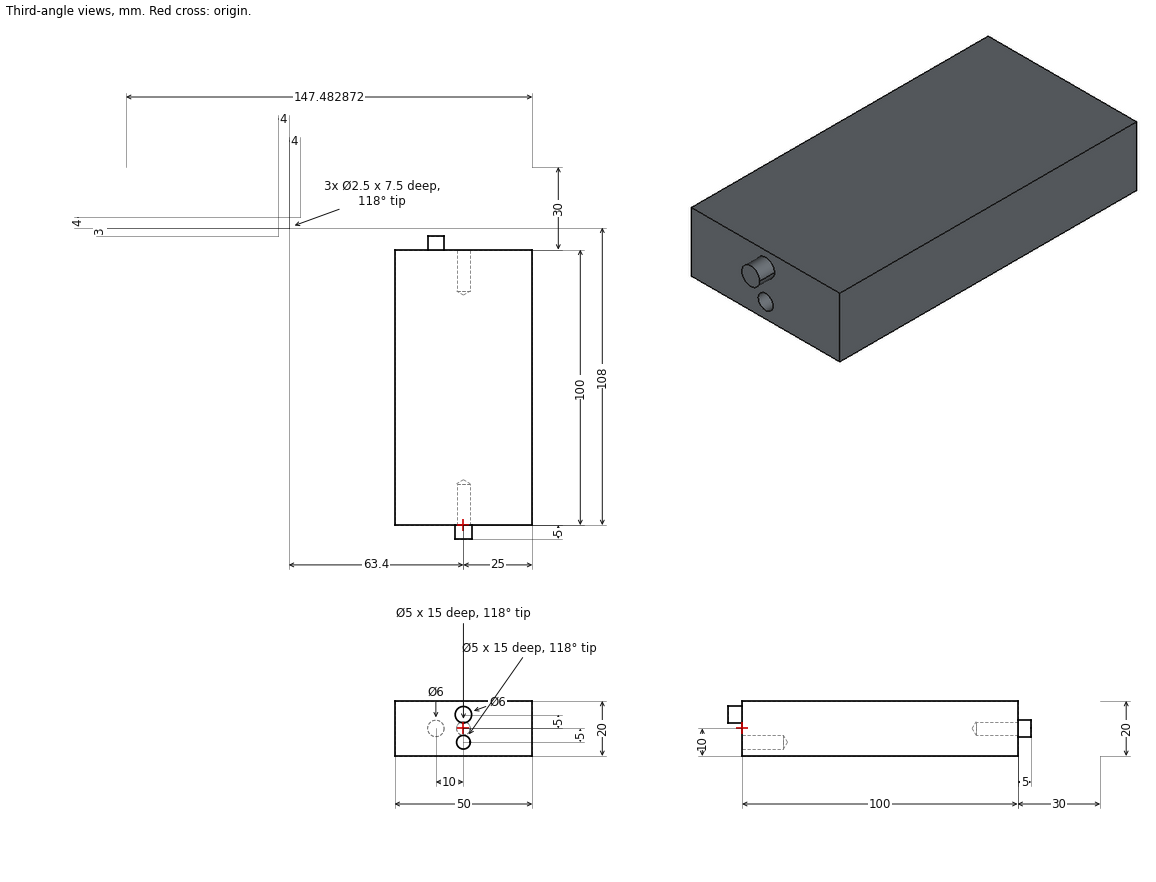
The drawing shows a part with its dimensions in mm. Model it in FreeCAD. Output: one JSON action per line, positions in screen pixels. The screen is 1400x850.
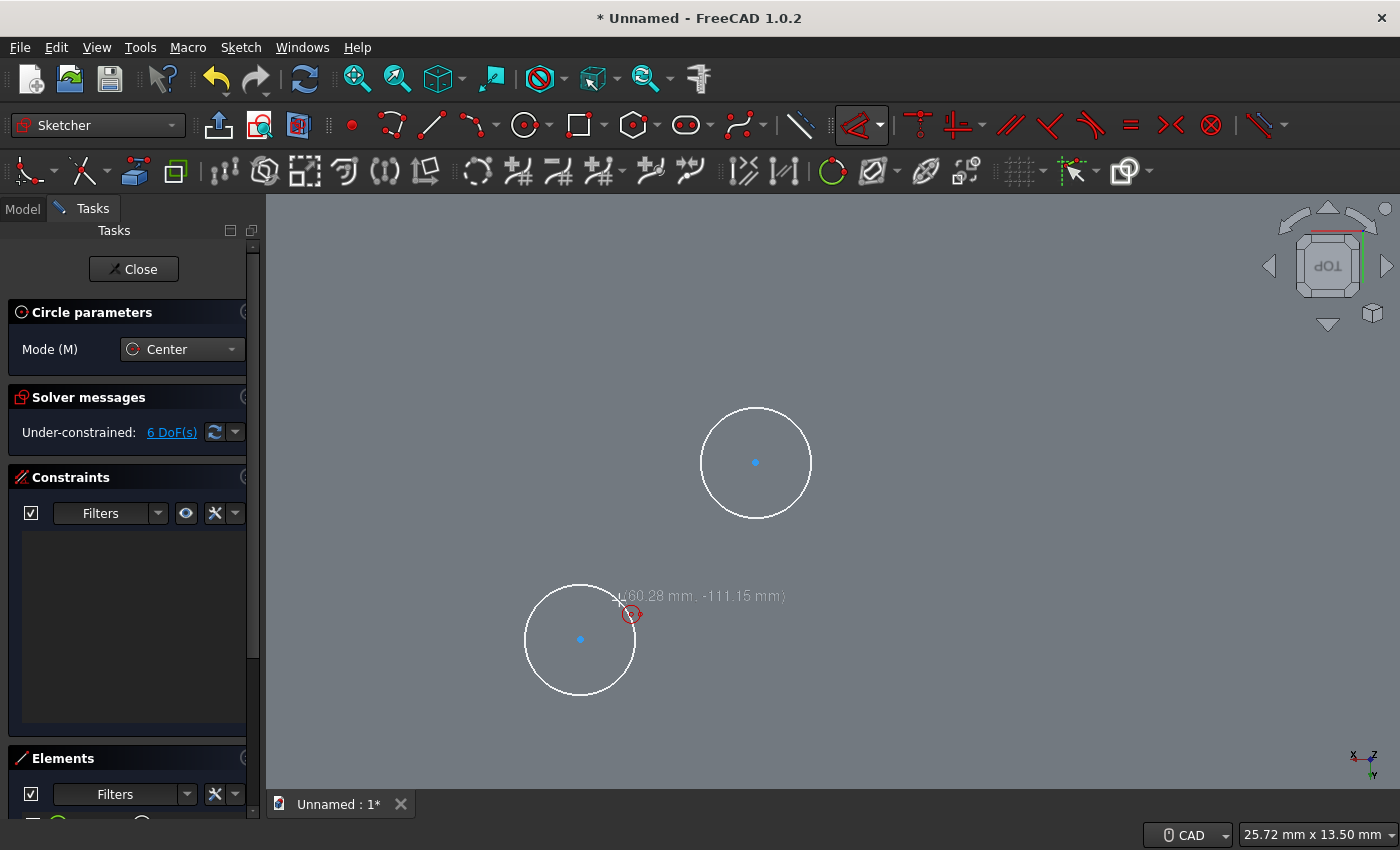
{"action": "left_click", "coordinate": [933, 330]}
{"action": "left_click", "coordinate": [972, 291]}
{"action": "key", "text": "Escape"}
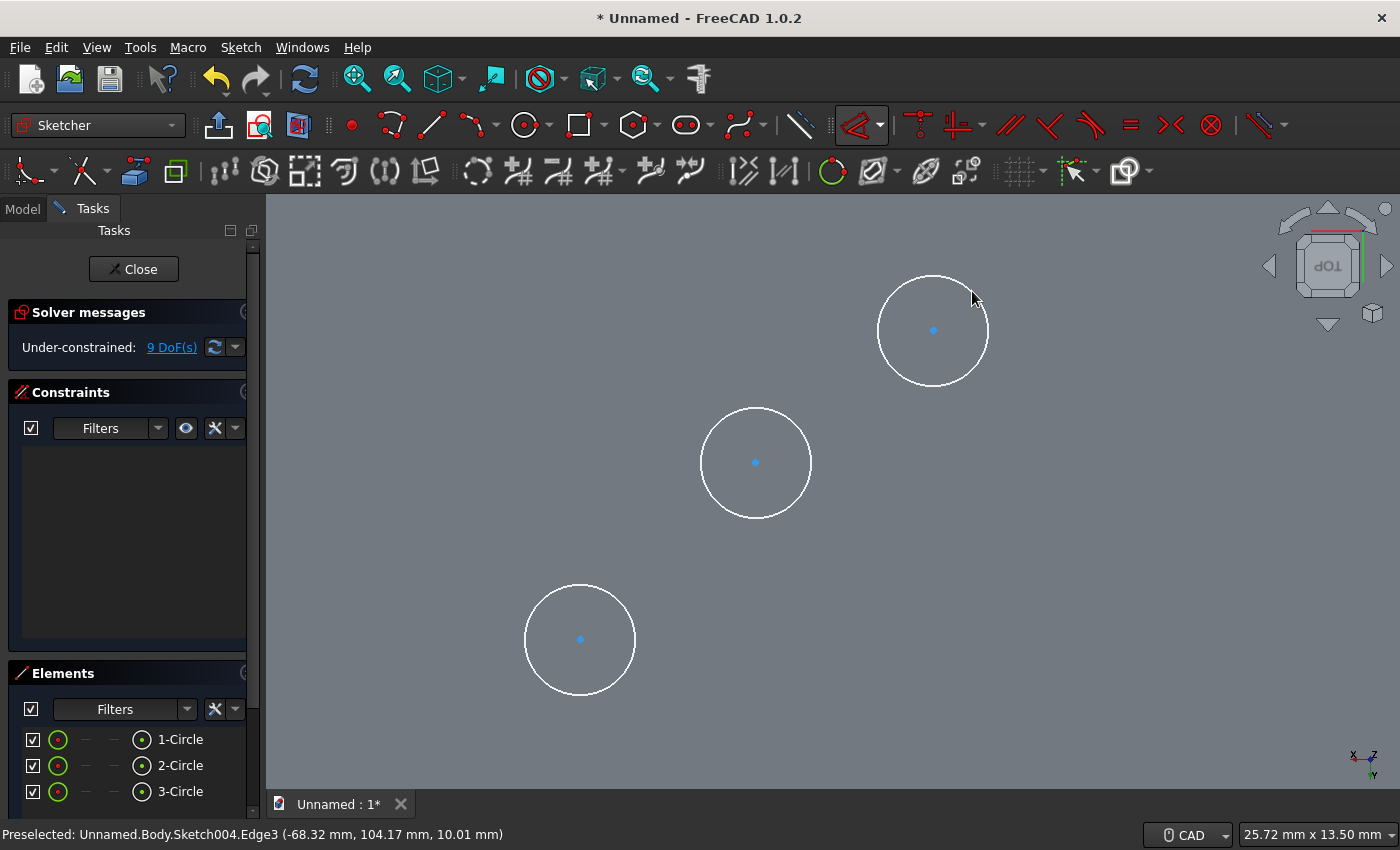
{"action": "left_click", "coordinate": [795, 424]}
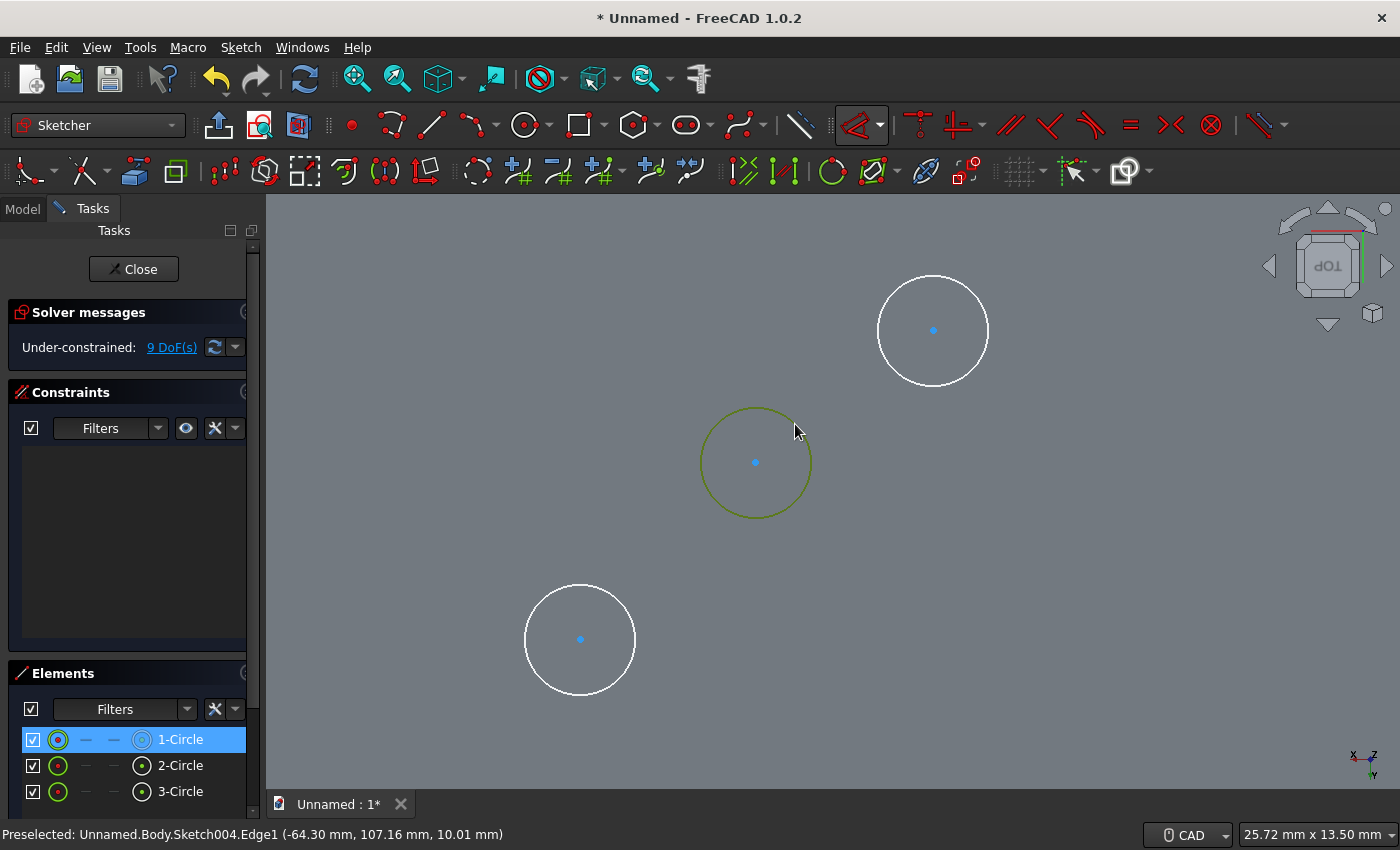
{"action": "left_click", "coordinate": [619, 601]}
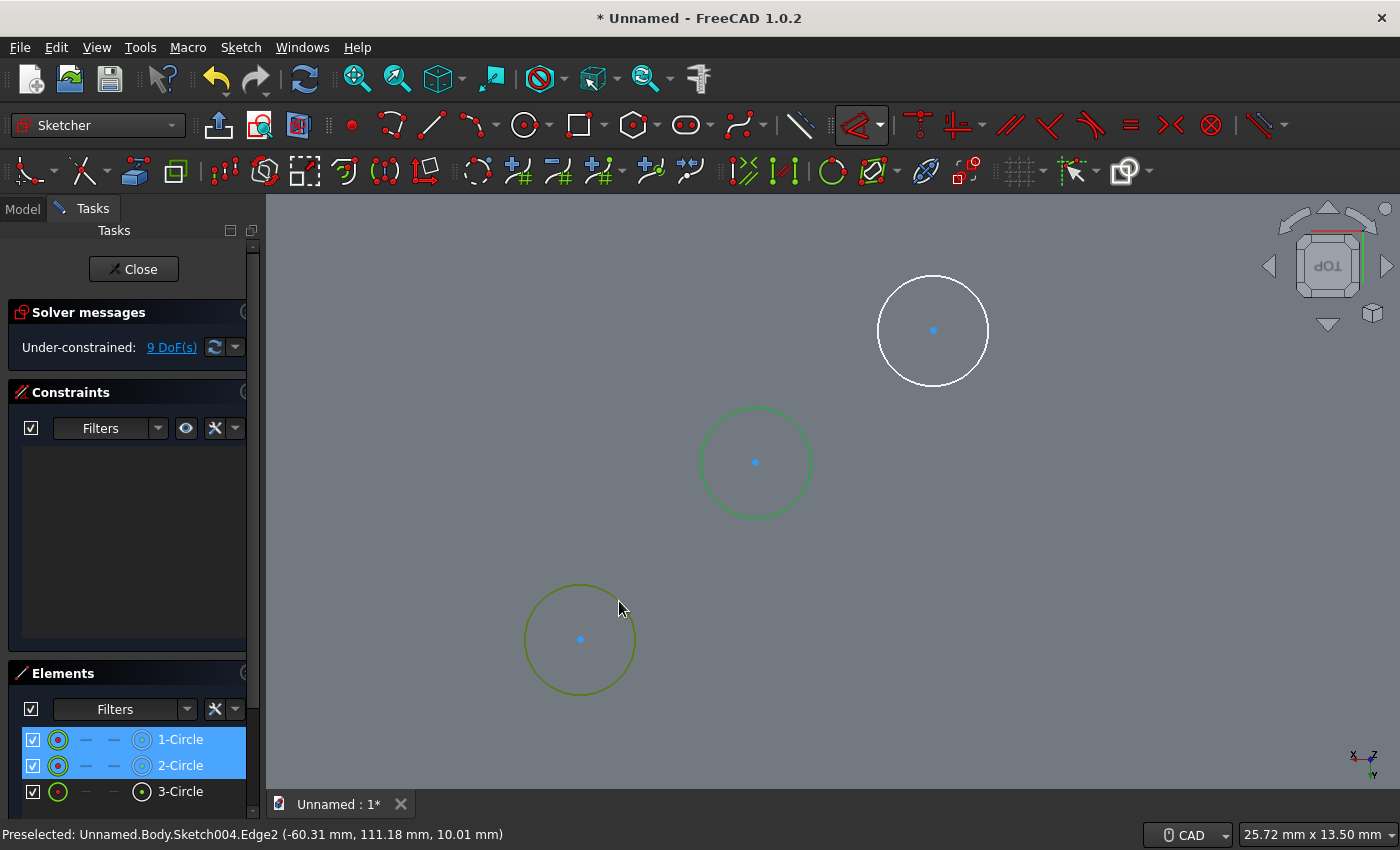
{"action": "left_click", "coordinate": [972, 292]}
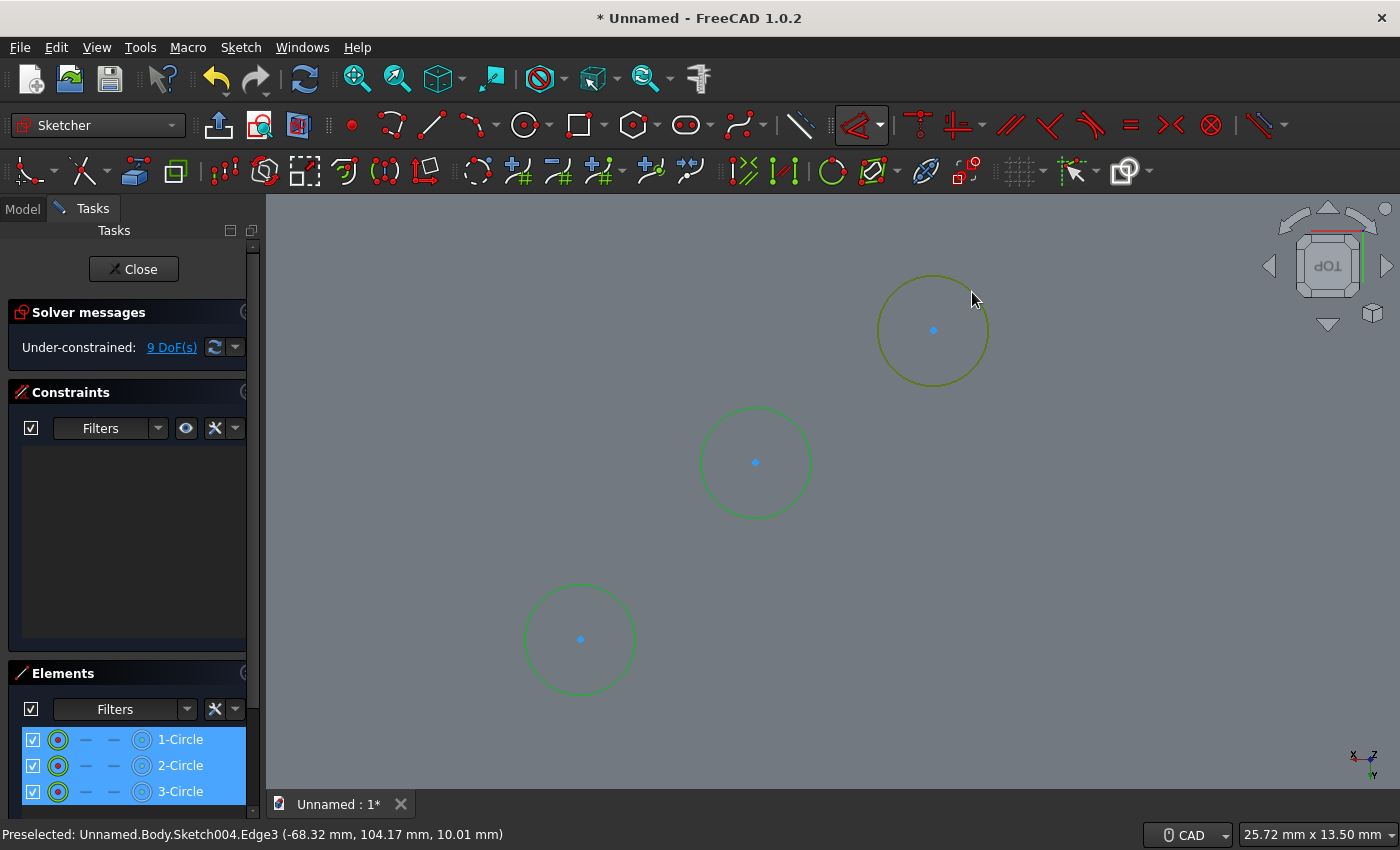
{"action": "left_click", "coordinate": [1132, 126]}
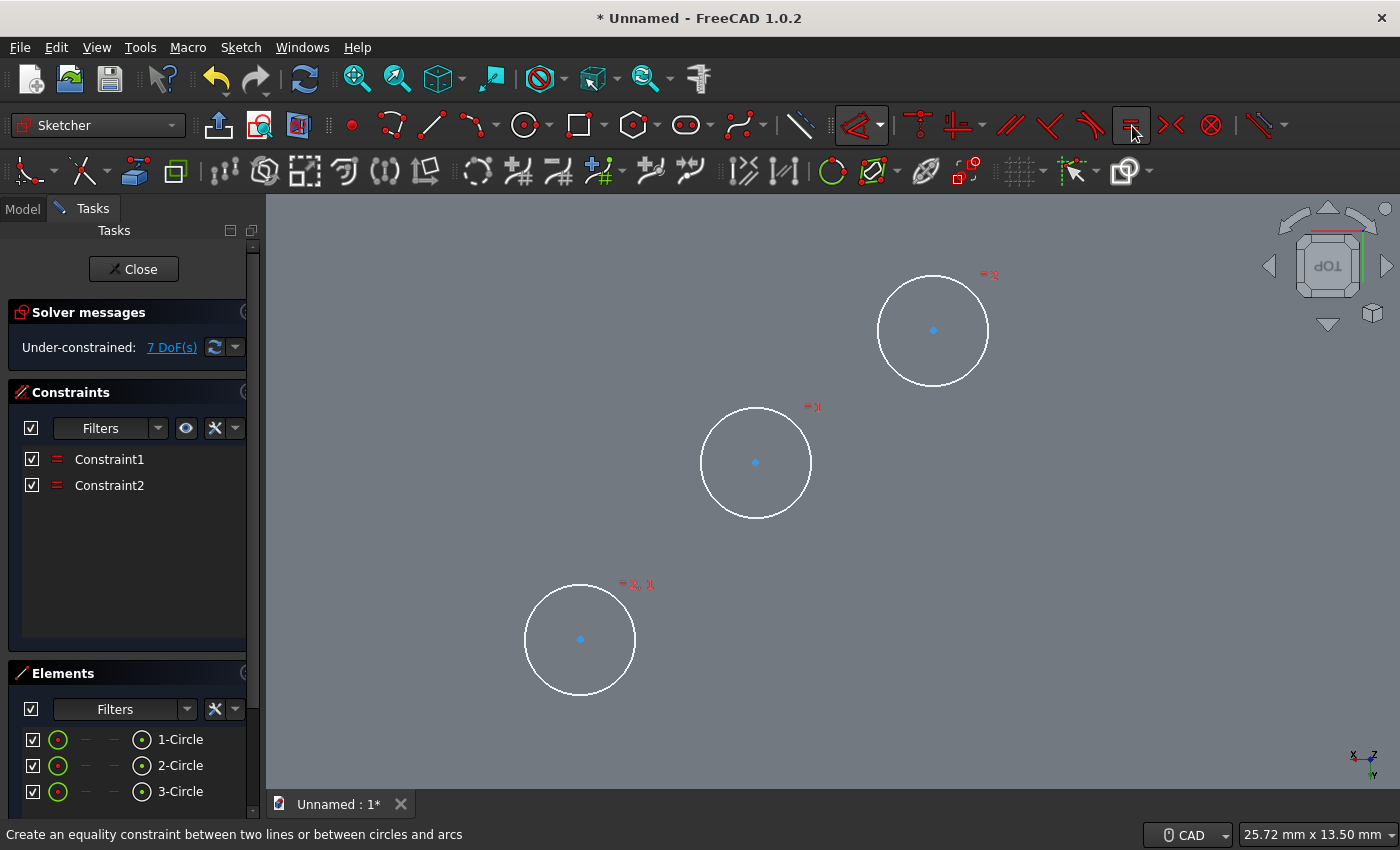
{"action": "left_click", "coordinate": [795, 424]}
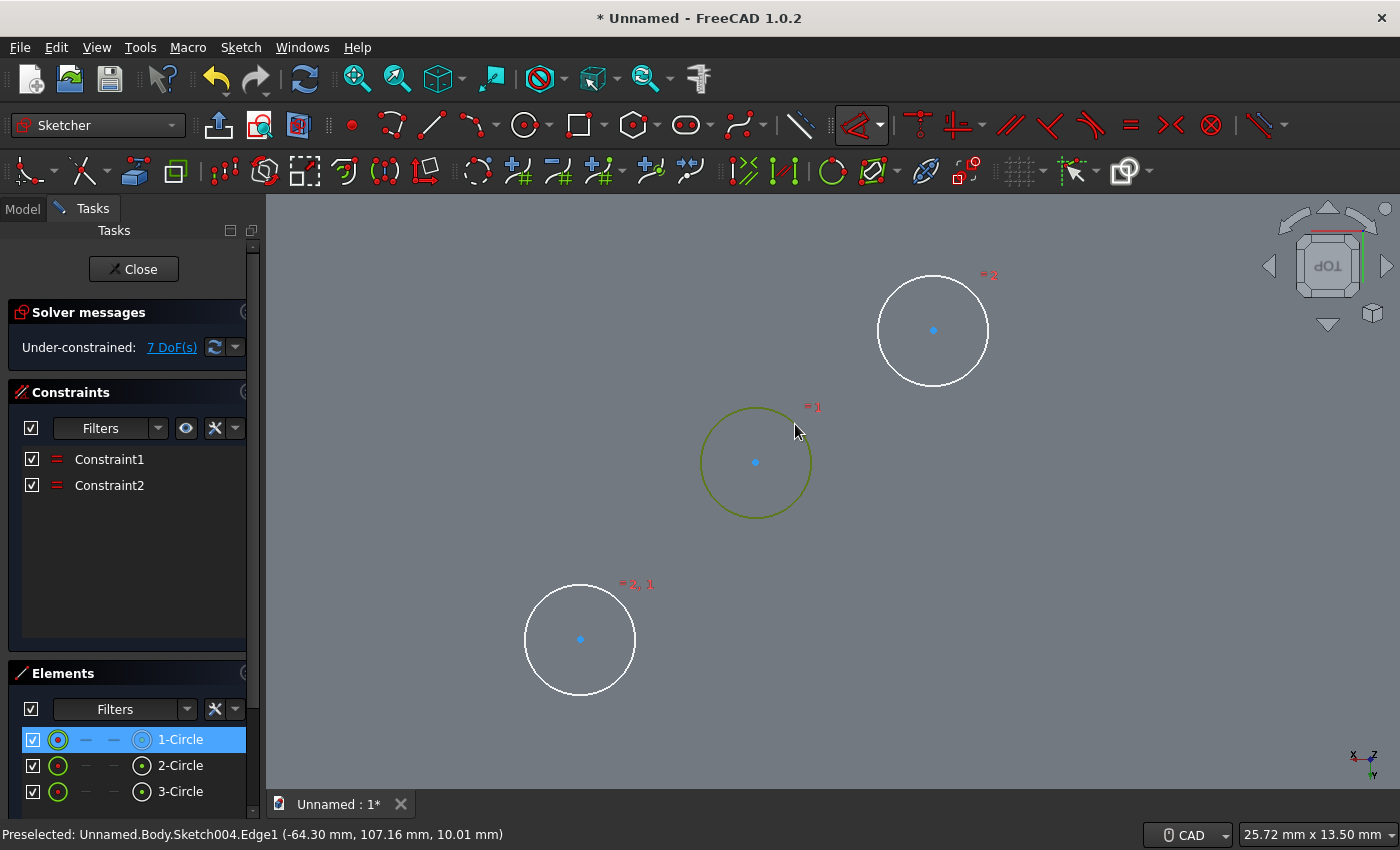
{"action": "key", "text": "k o"}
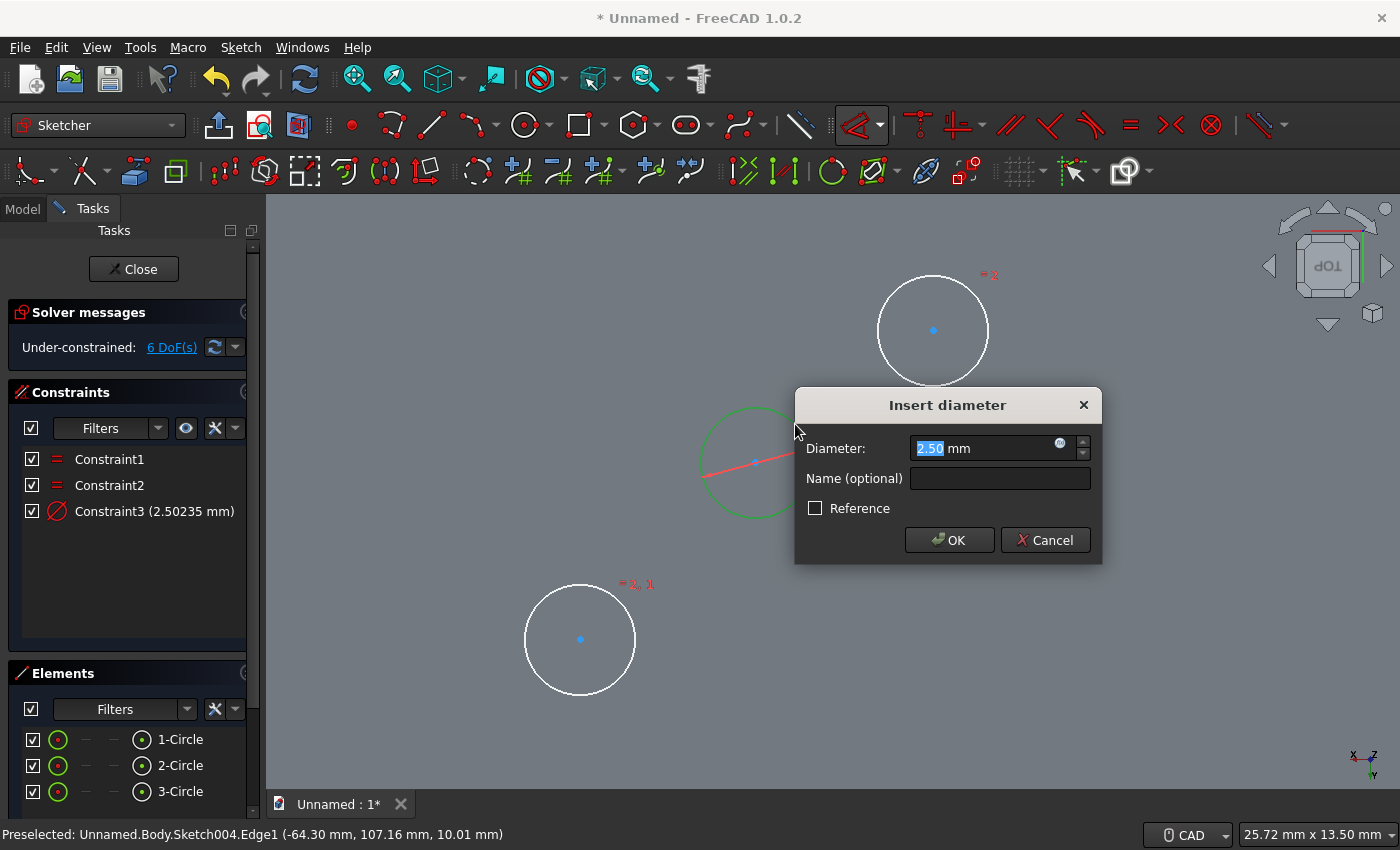
{"action": "type", "text": "2.5"}
{"action": "key", "text": "Return"}